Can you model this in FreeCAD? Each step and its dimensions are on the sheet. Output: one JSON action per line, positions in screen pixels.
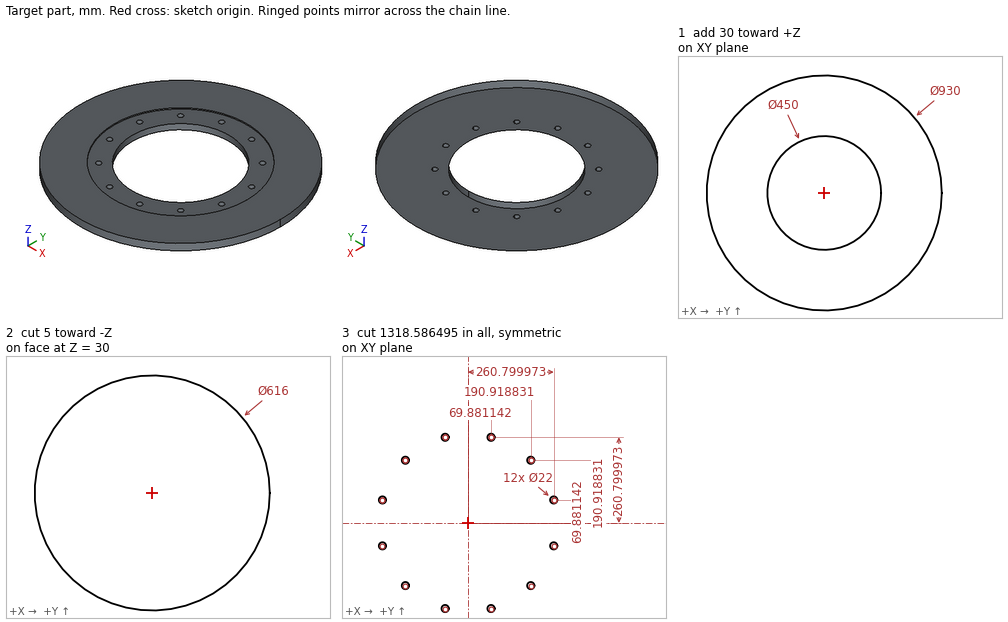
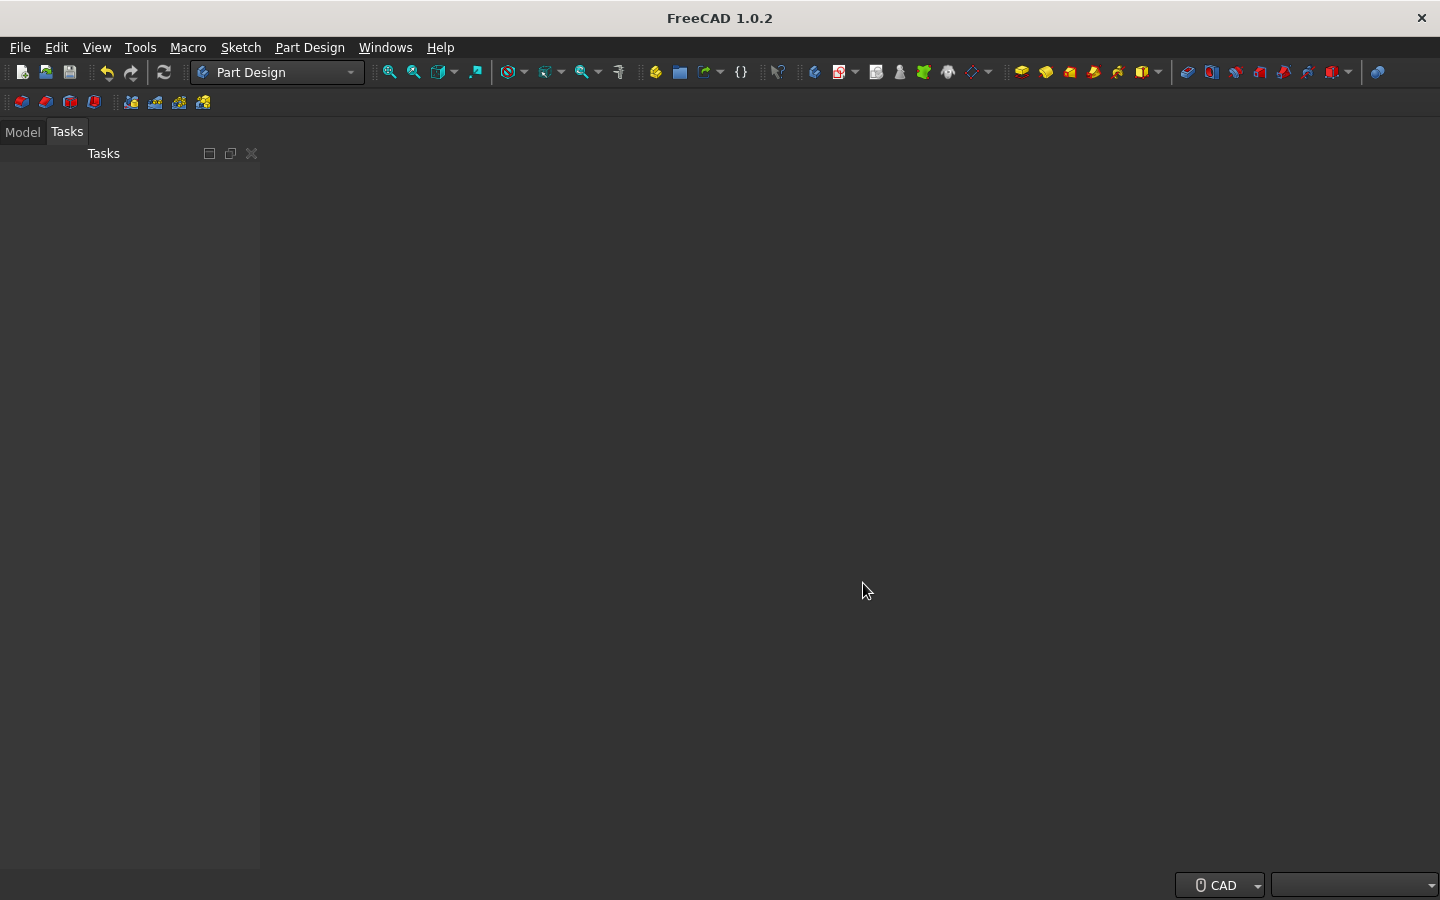
{"action": "left_click", "coordinate": [22, 72]}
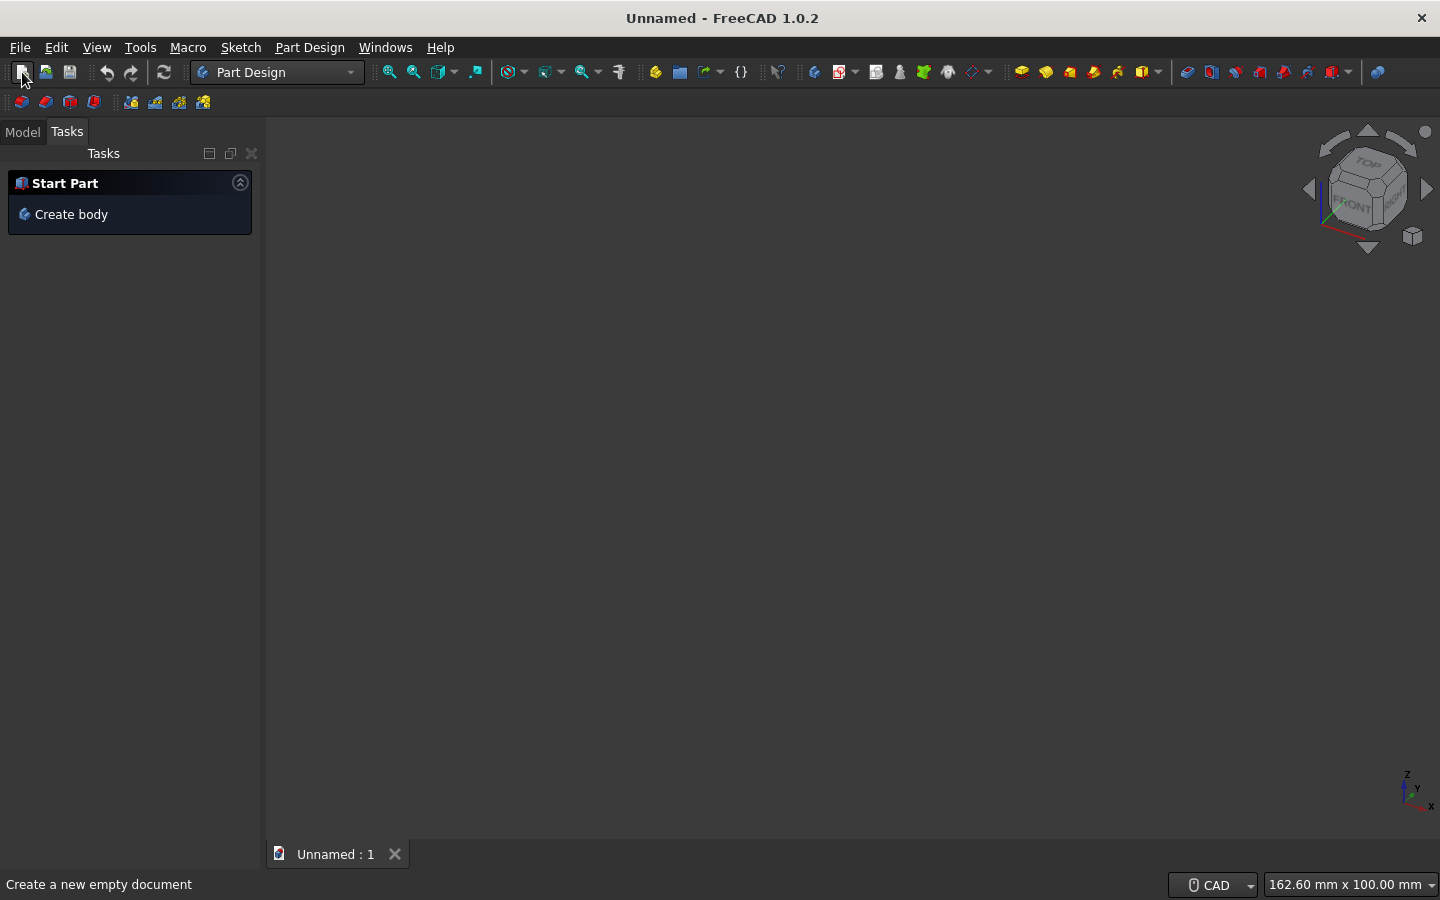
{"action": "left_click", "coordinate": [840, 72]}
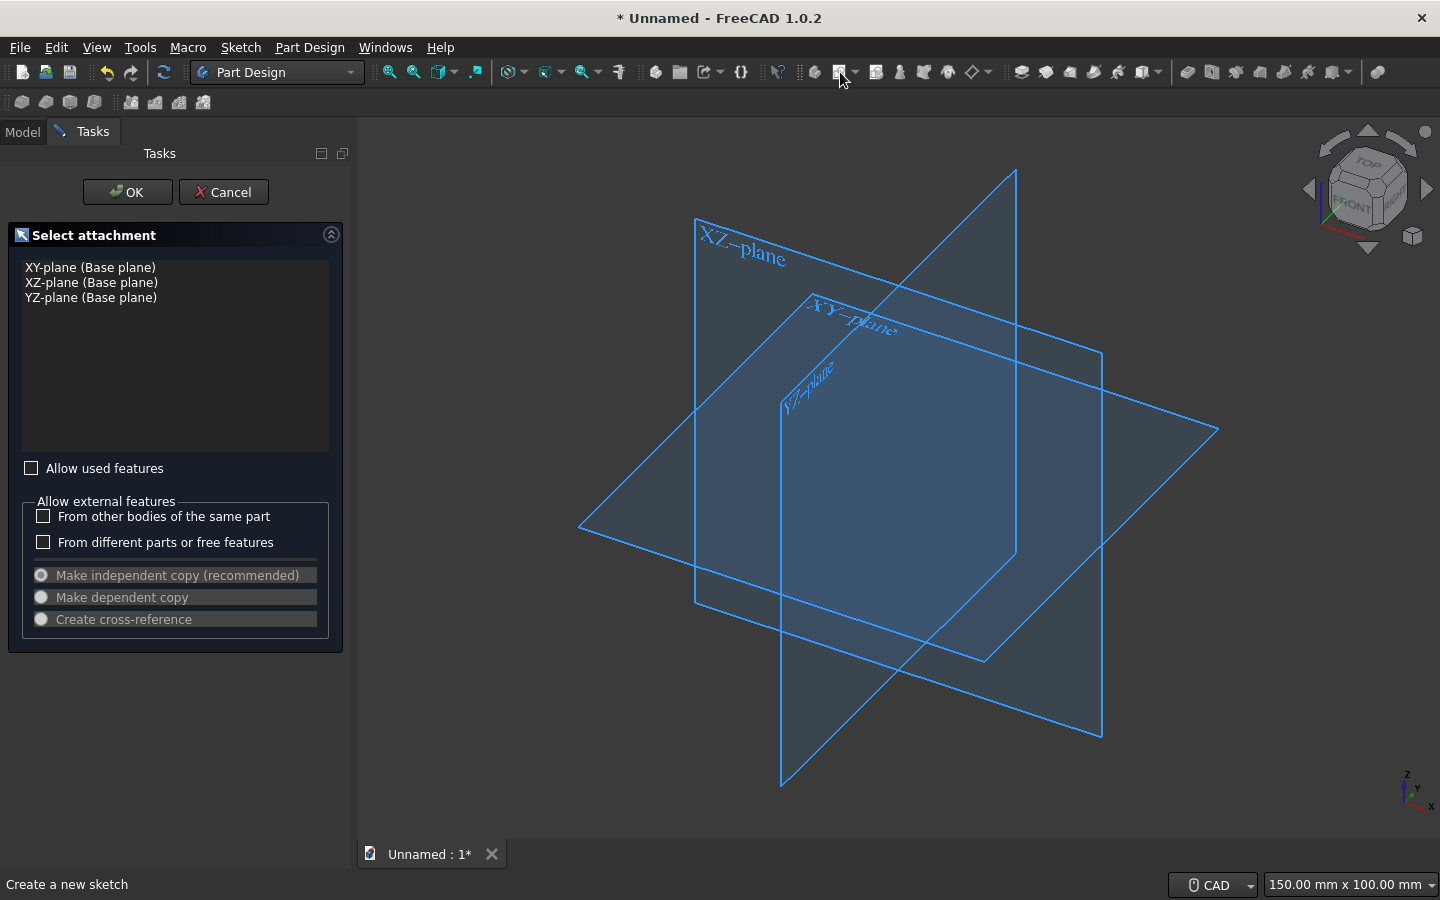
{"action": "left_click", "coordinate": [82, 268]}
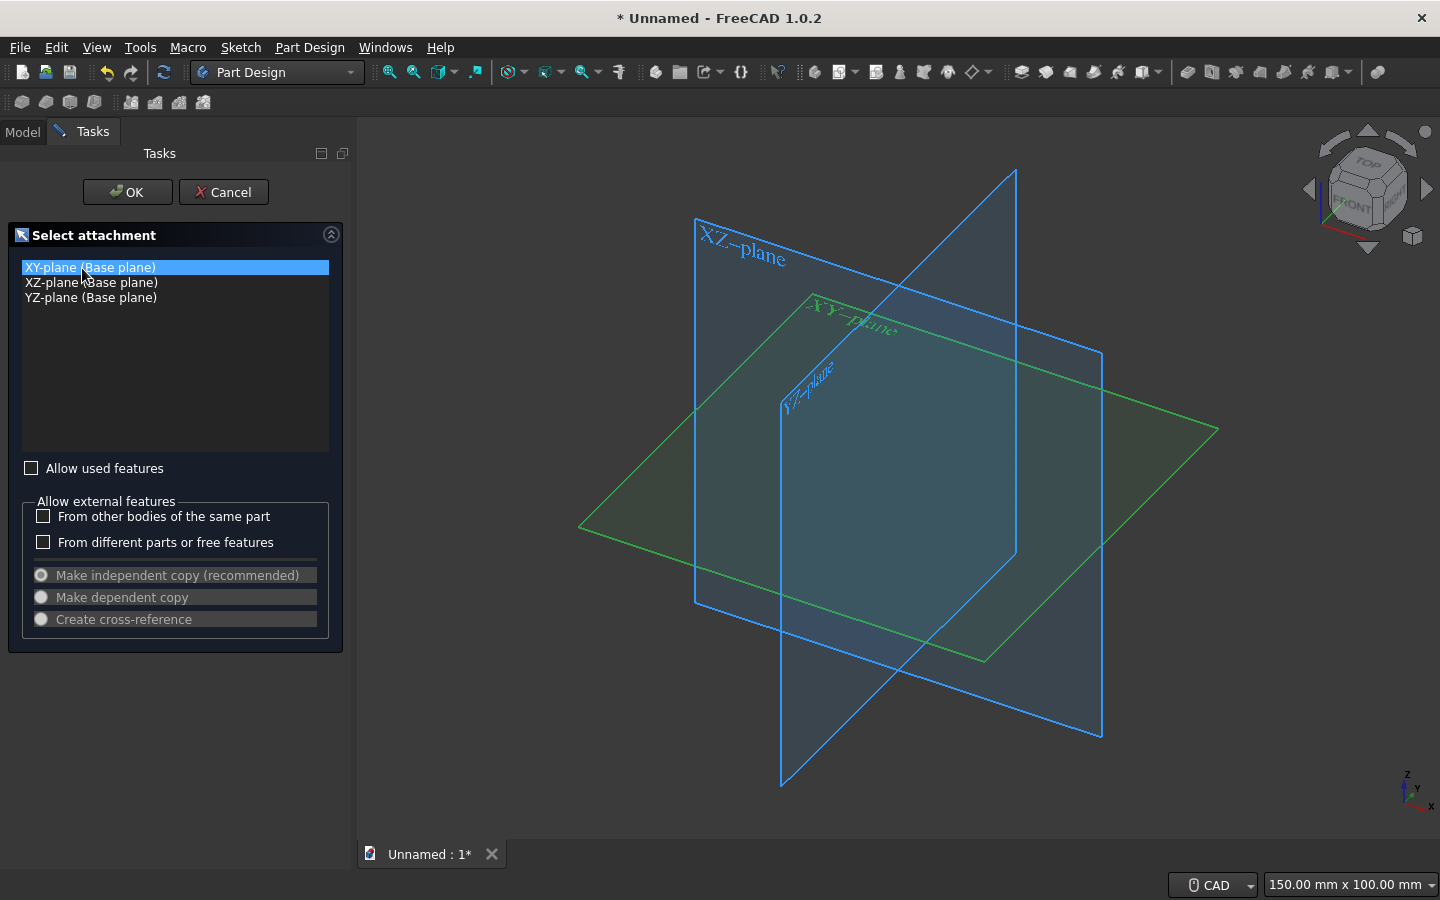
{"action": "left_click", "coordinate": [128, 192]}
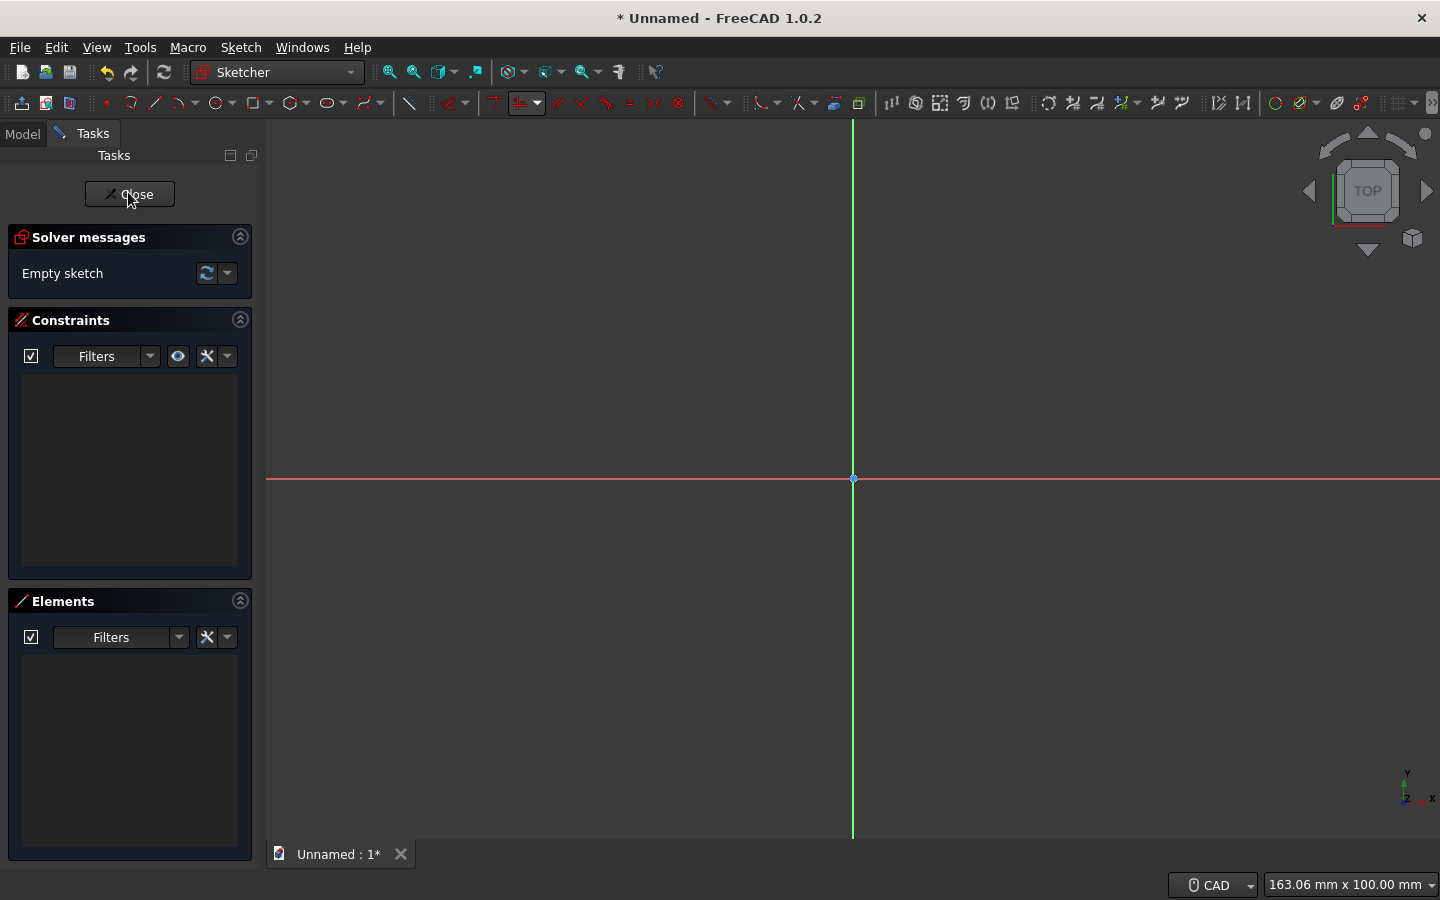
{"action": "scroll", "coordinate": [779, 479], "scroll_direction": "down", "scroll_amount": 13}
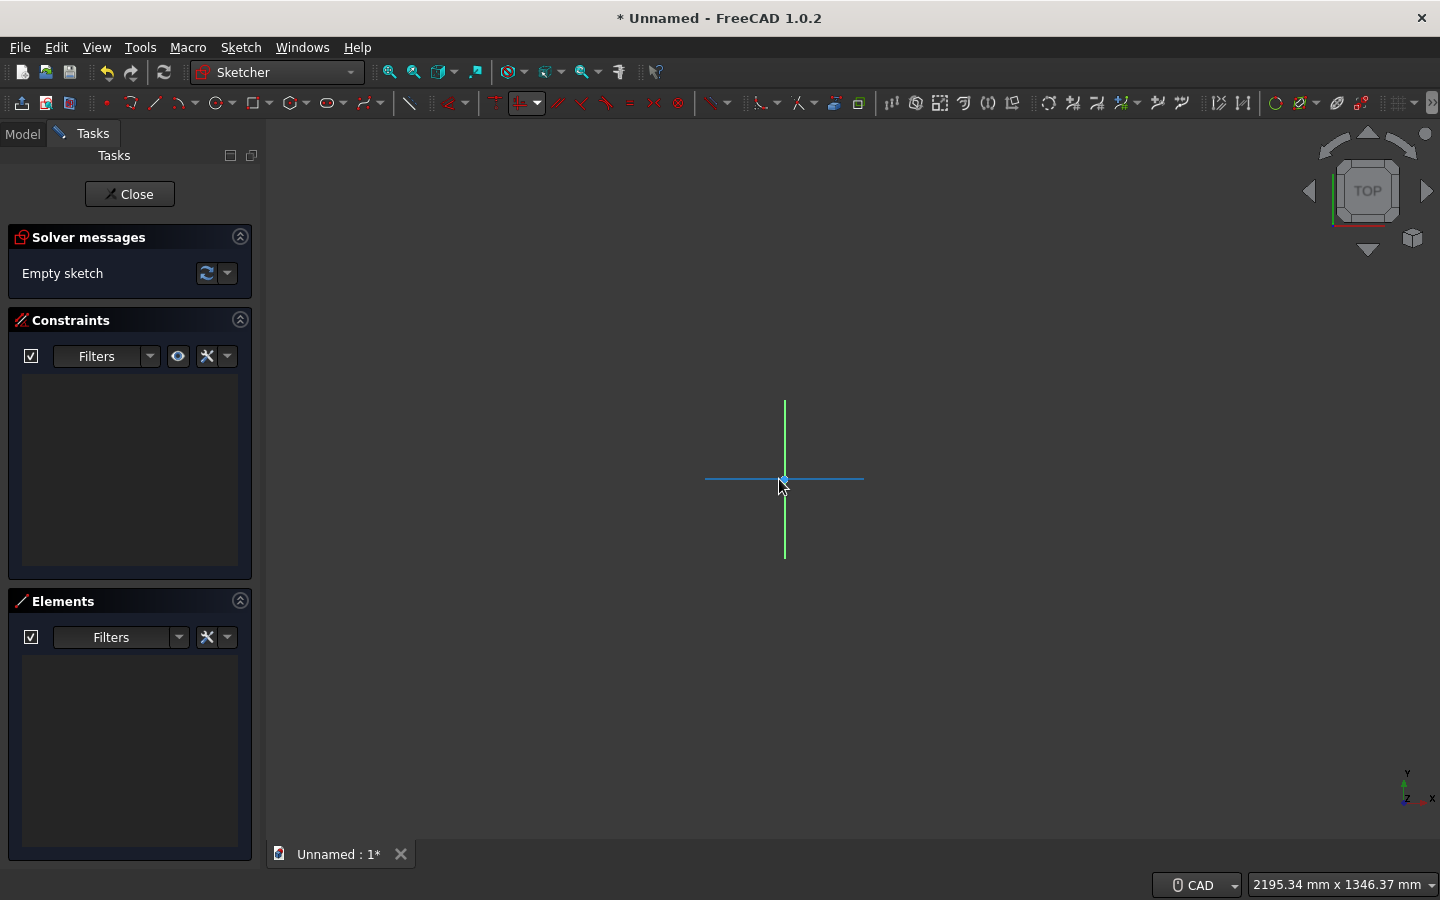
{"action": "left_click", "coordinate": [216, 104]}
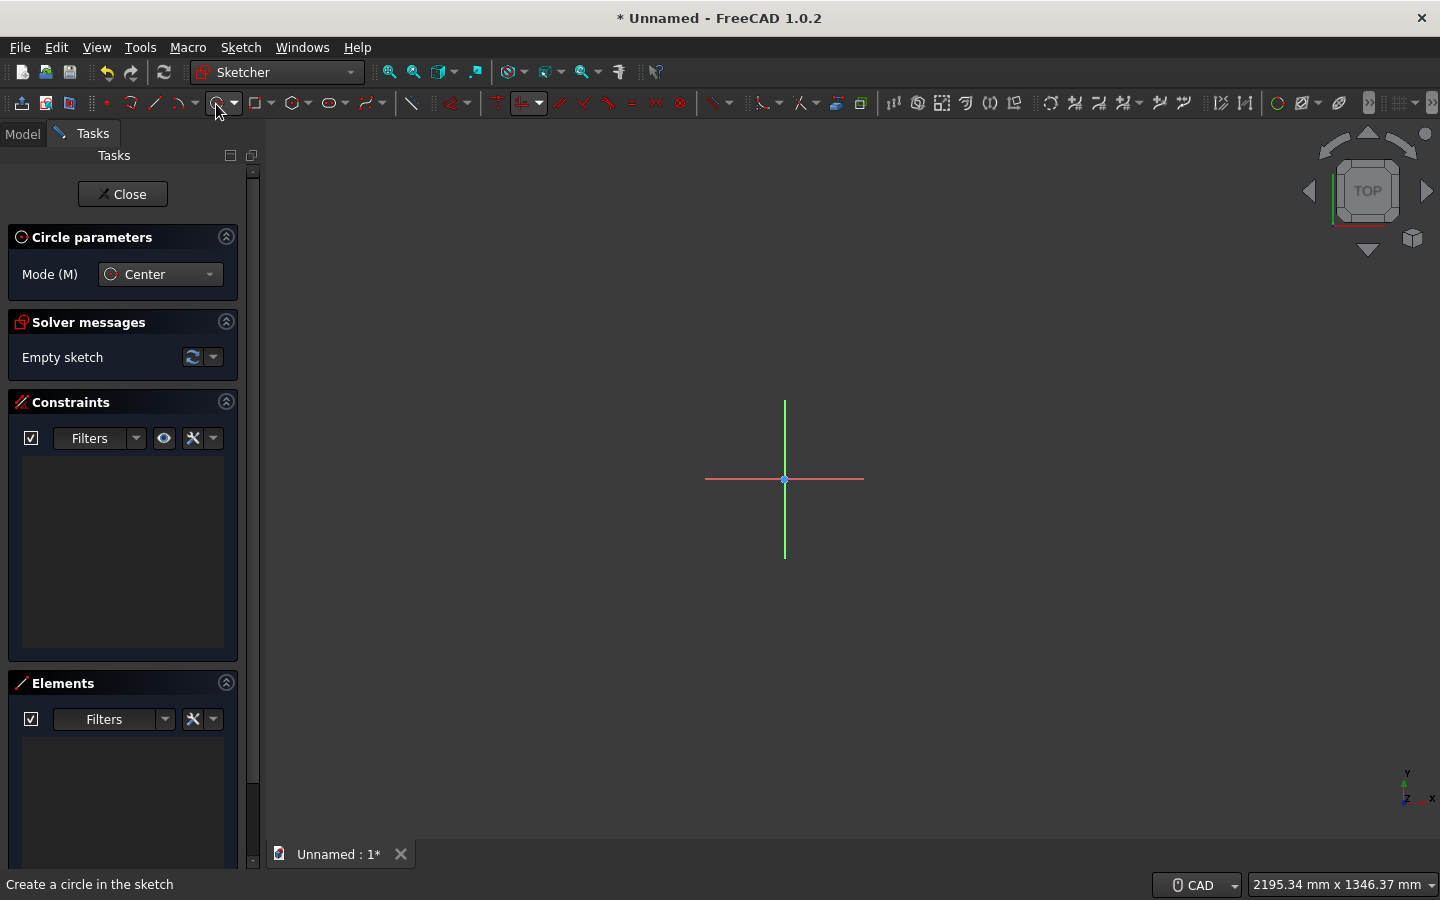
{"action": "left_click", "coordinate": [785, 479]}
{"action": "mouse_move", "coordinate": [961, 304]}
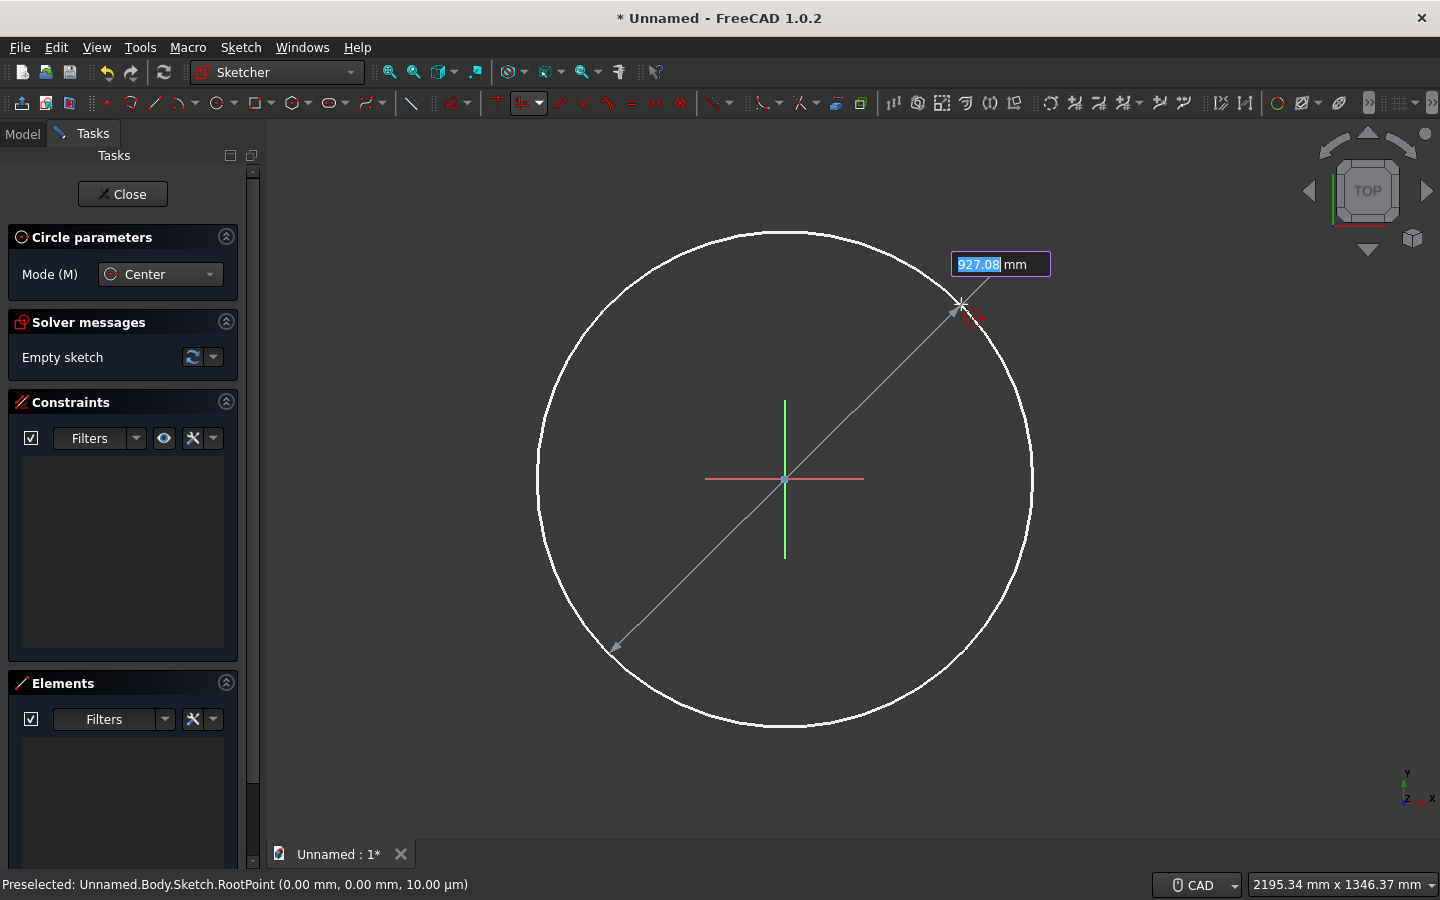
{"action": "type", "text": "930"}
{"action": "key", "text": "Return"}